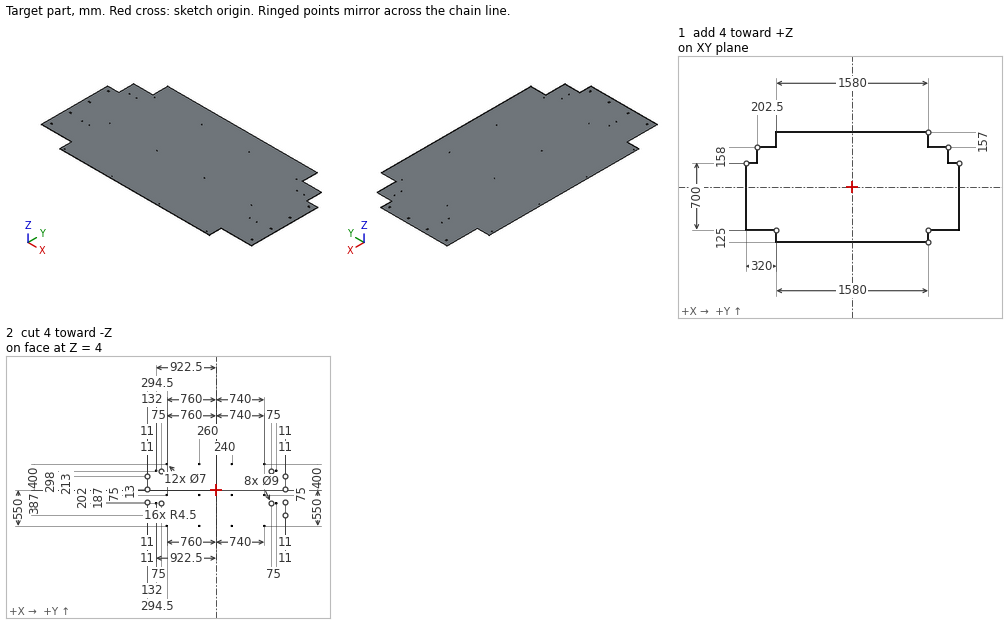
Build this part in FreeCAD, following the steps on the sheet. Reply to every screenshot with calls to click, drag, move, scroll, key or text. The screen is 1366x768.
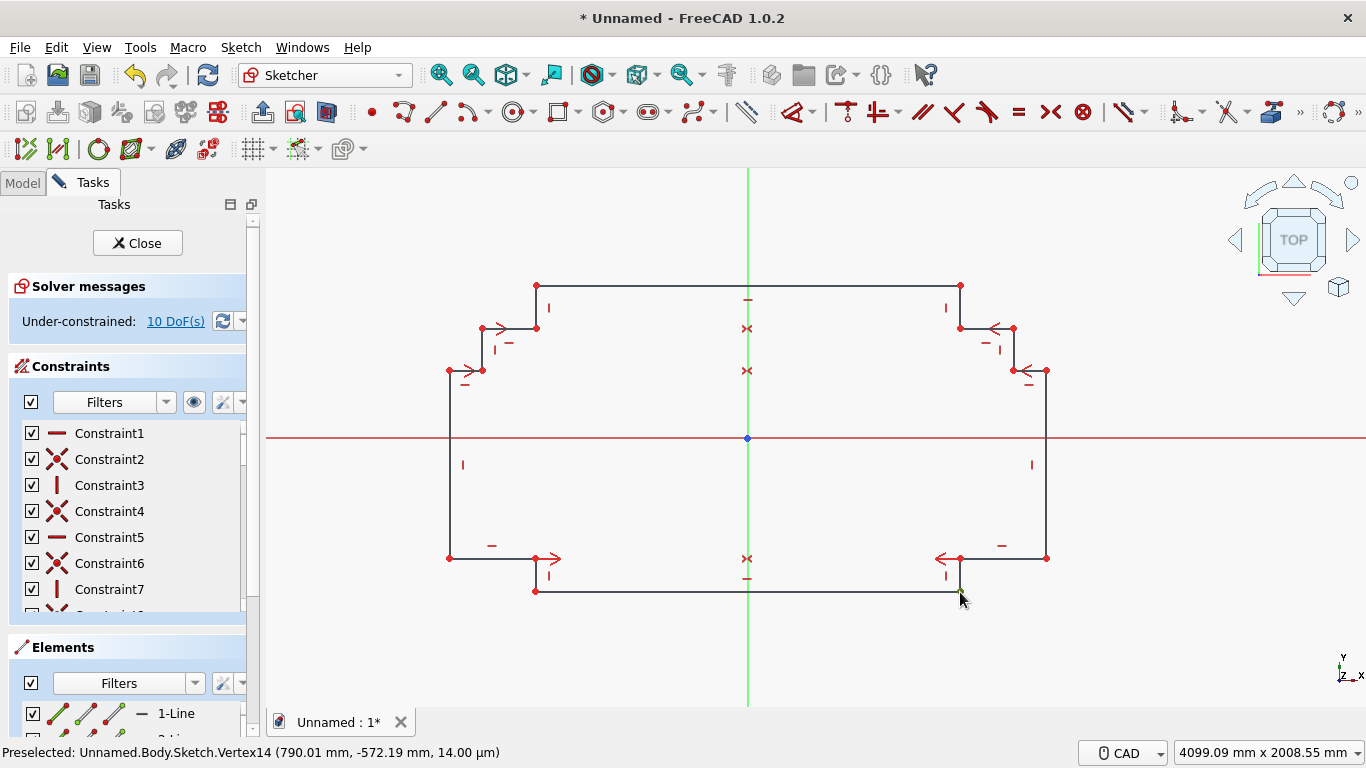
click(960, 286)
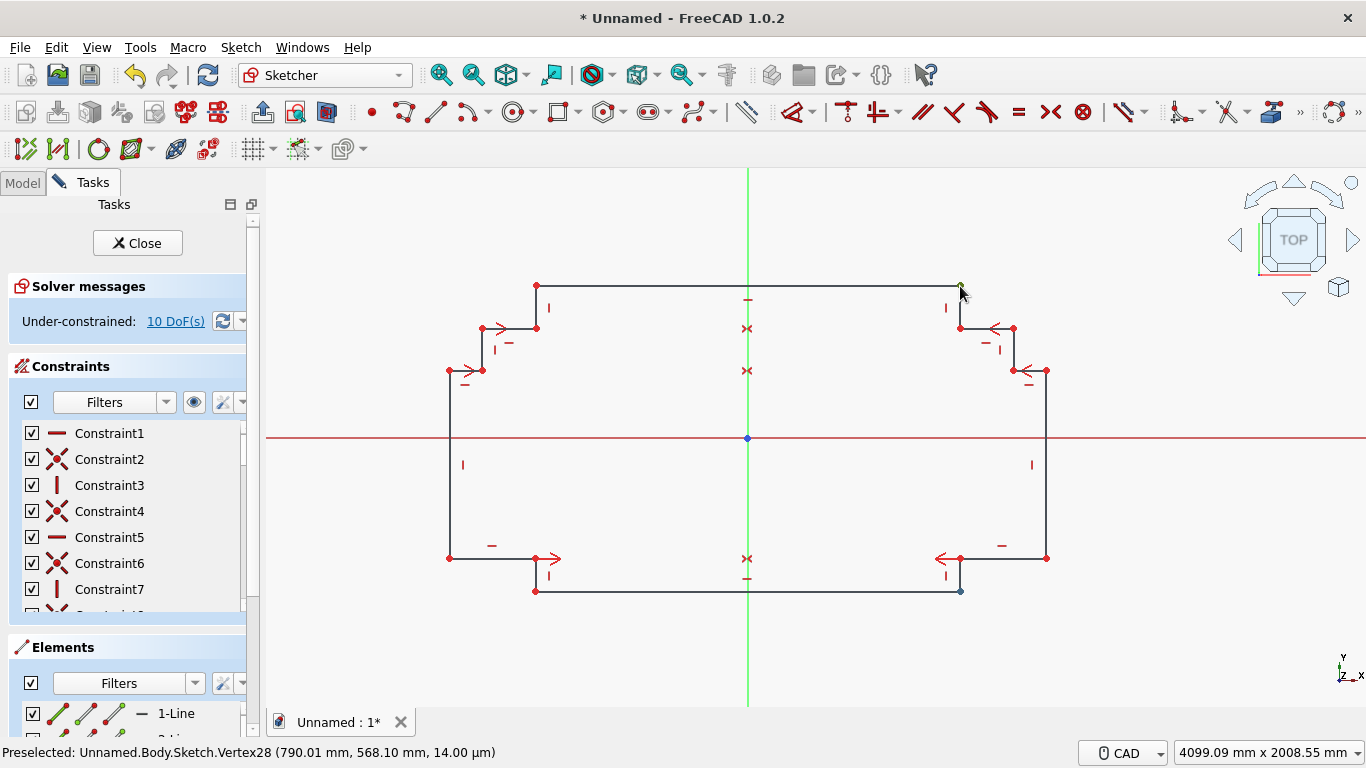
click(359, 438)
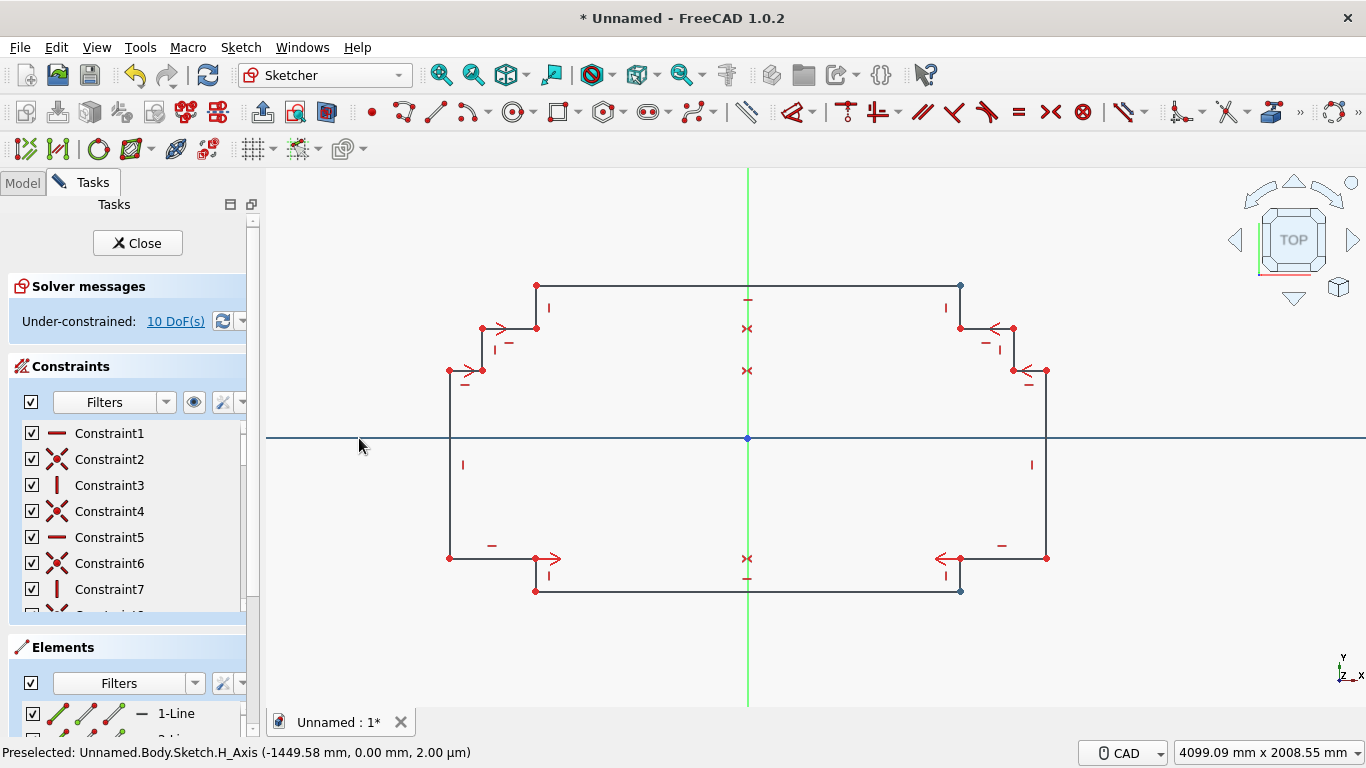
click(1052, 112)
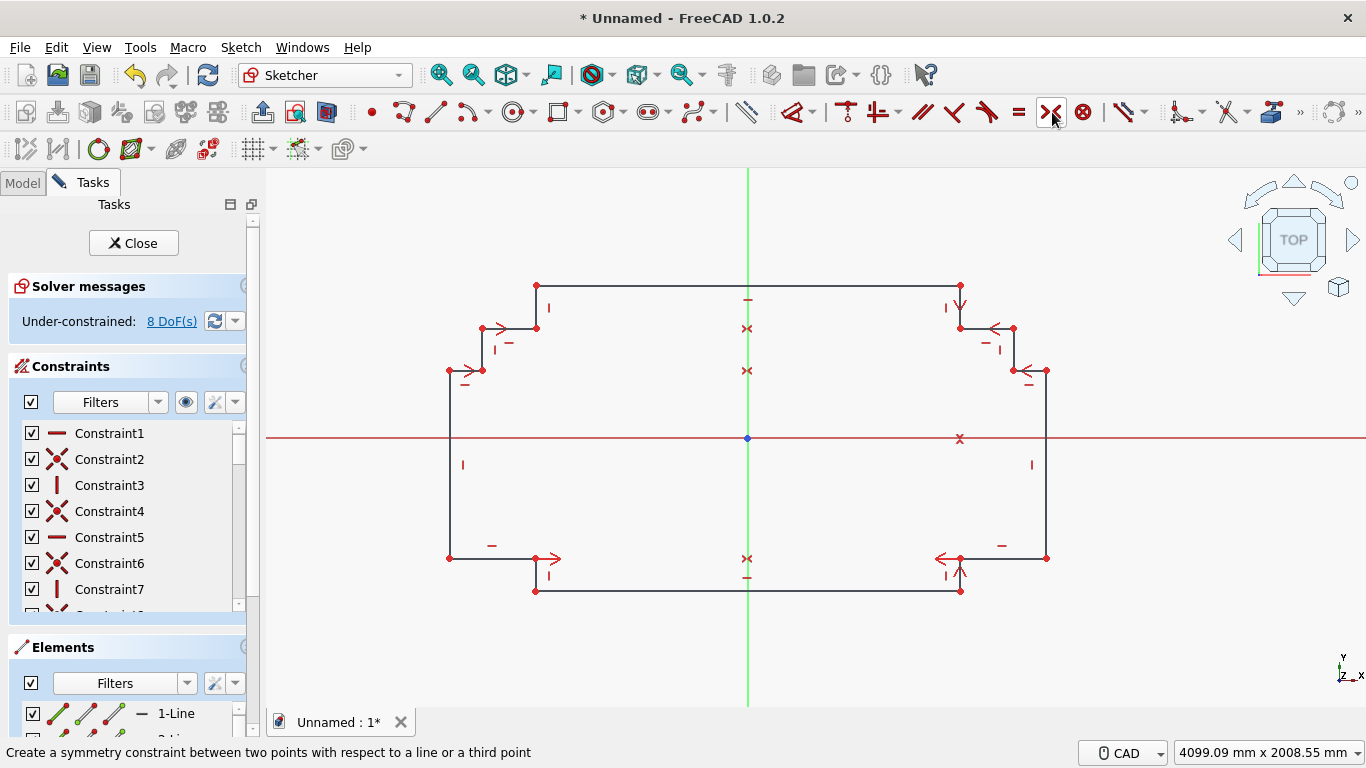
click(792, 112)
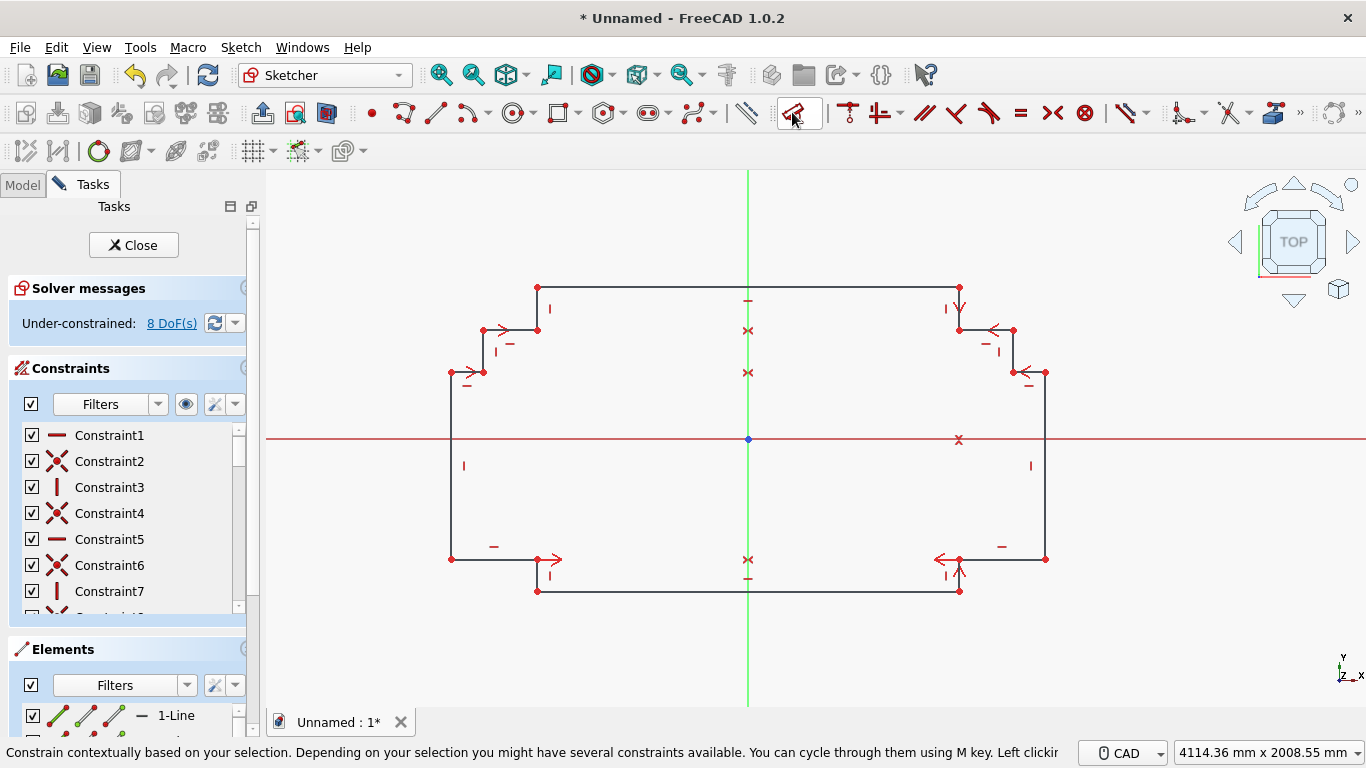
click(483, 343)
click(449, 351)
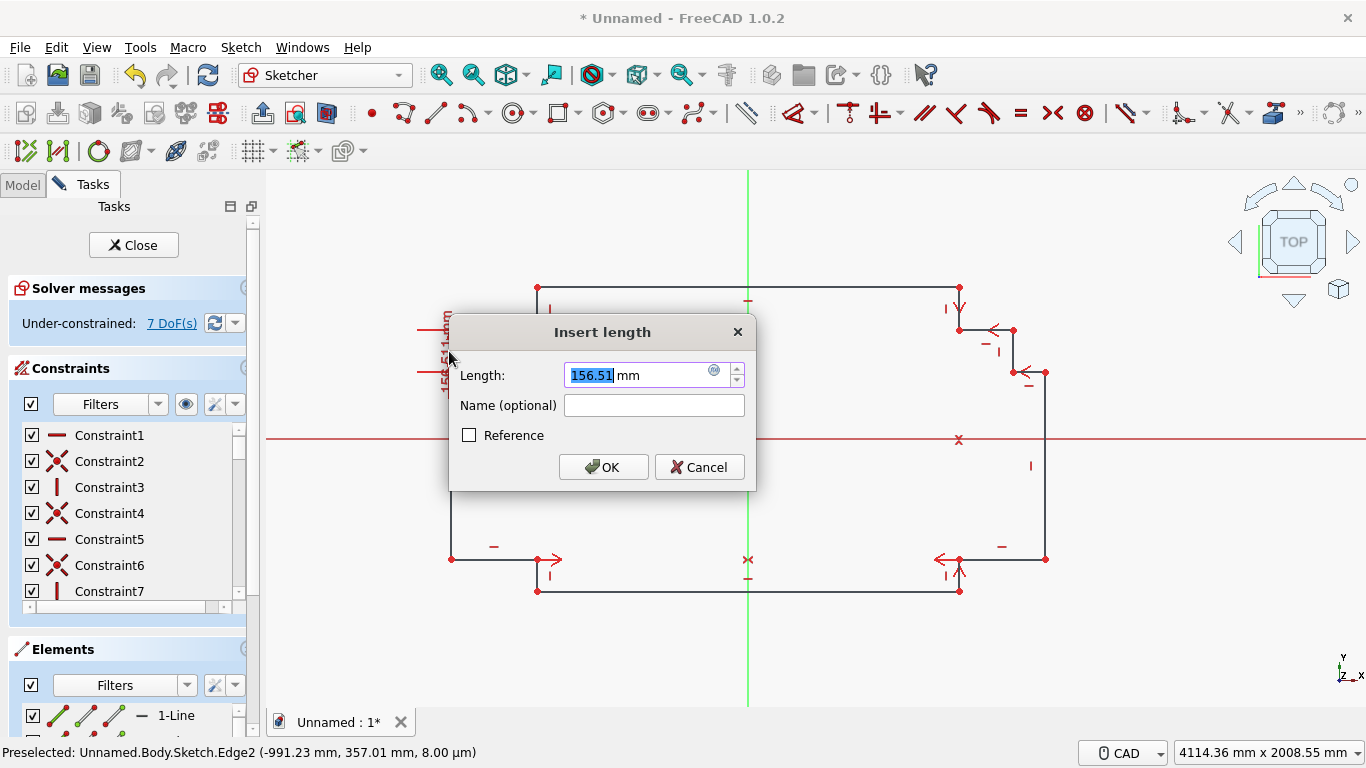
text(158)
key(Return)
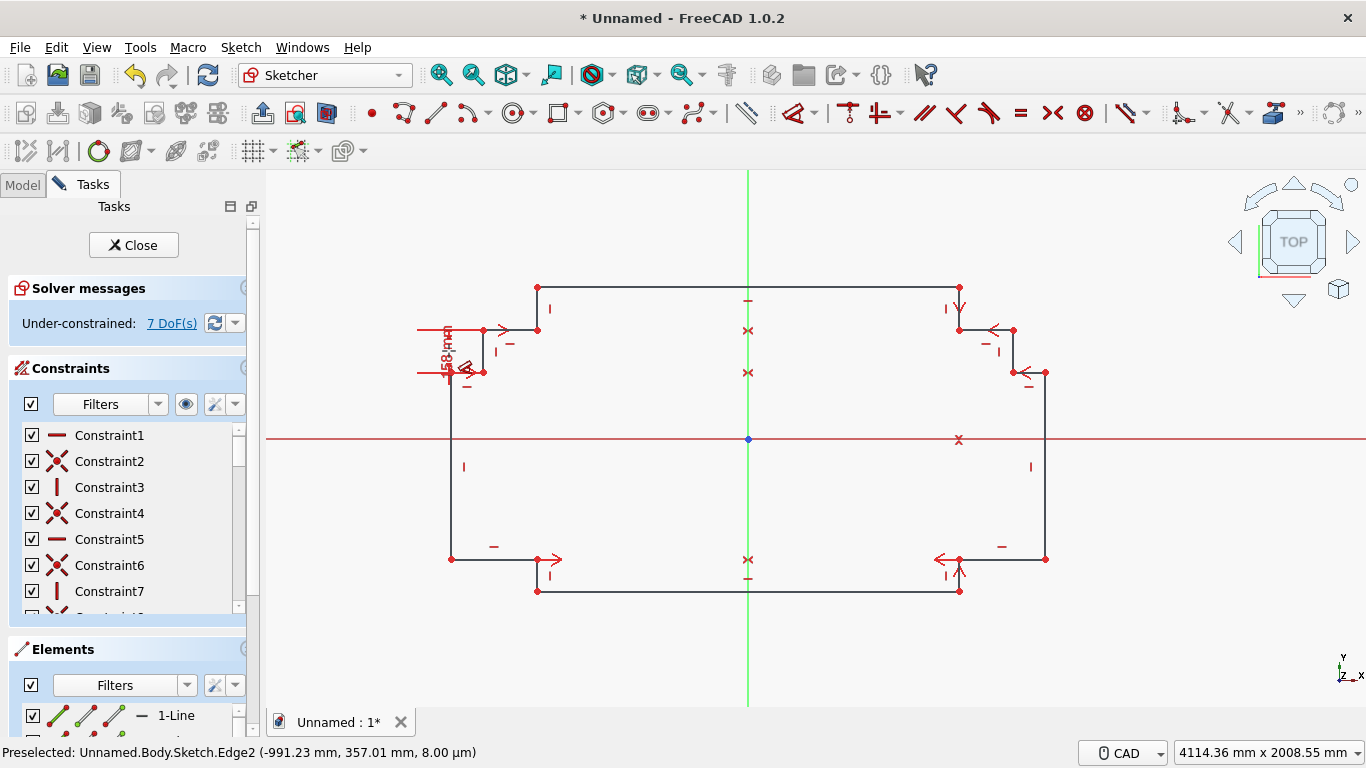
scroll(451, 429, up, 2)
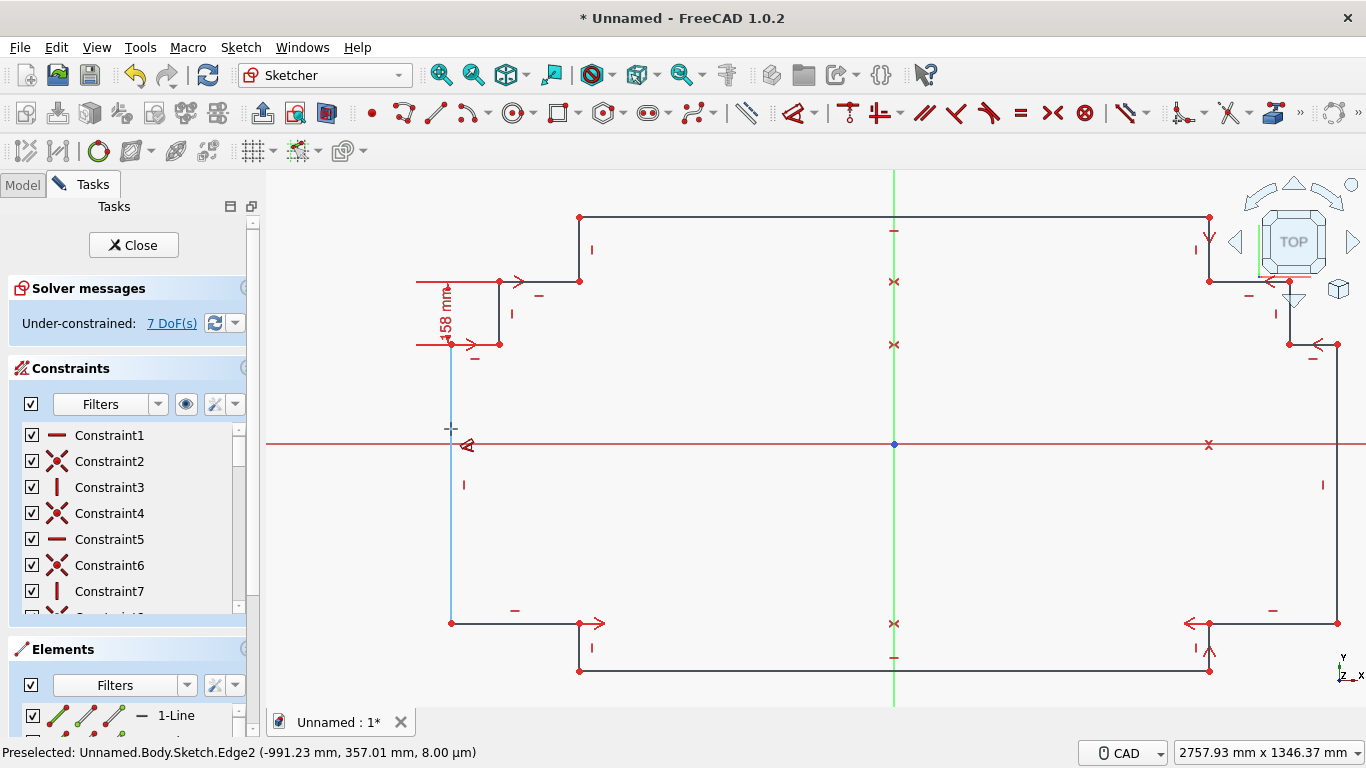
click(451, 428)
click(417, 484)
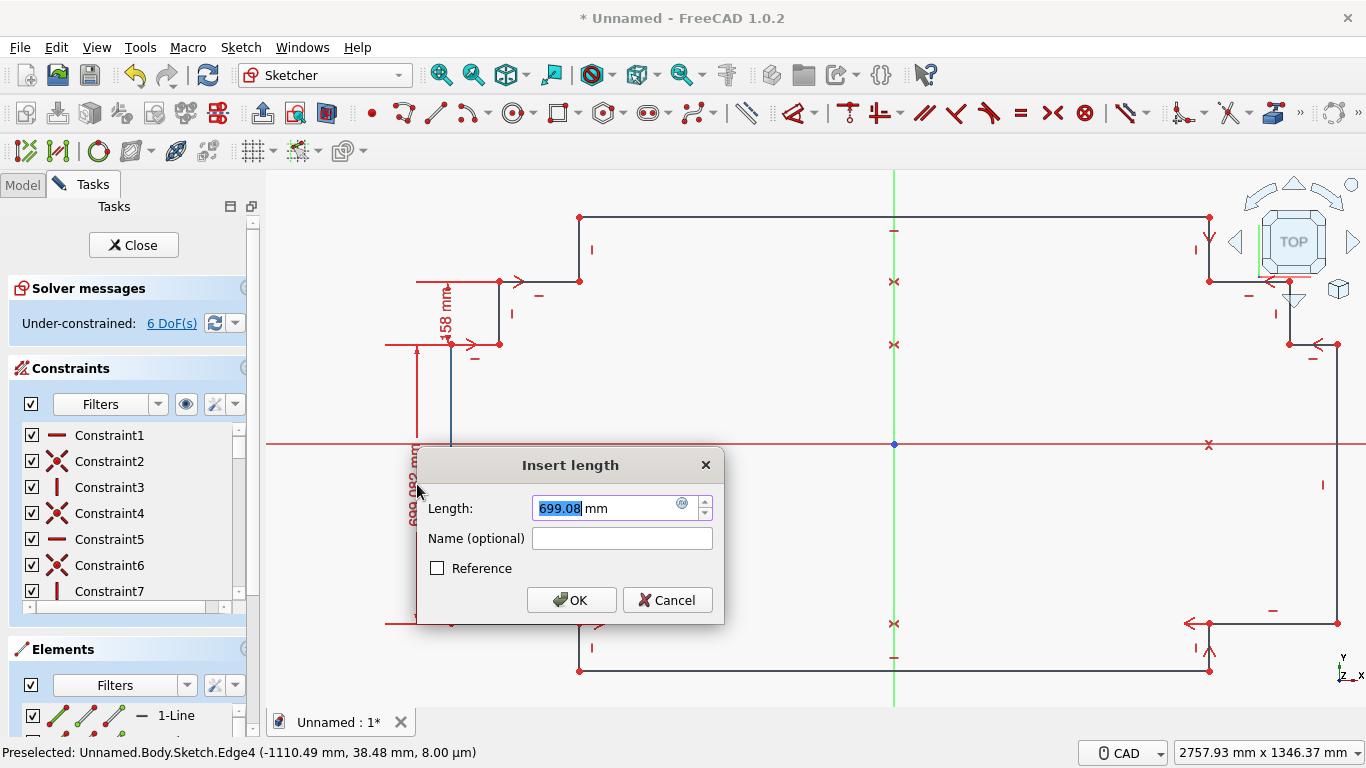
text(700)
key(Return)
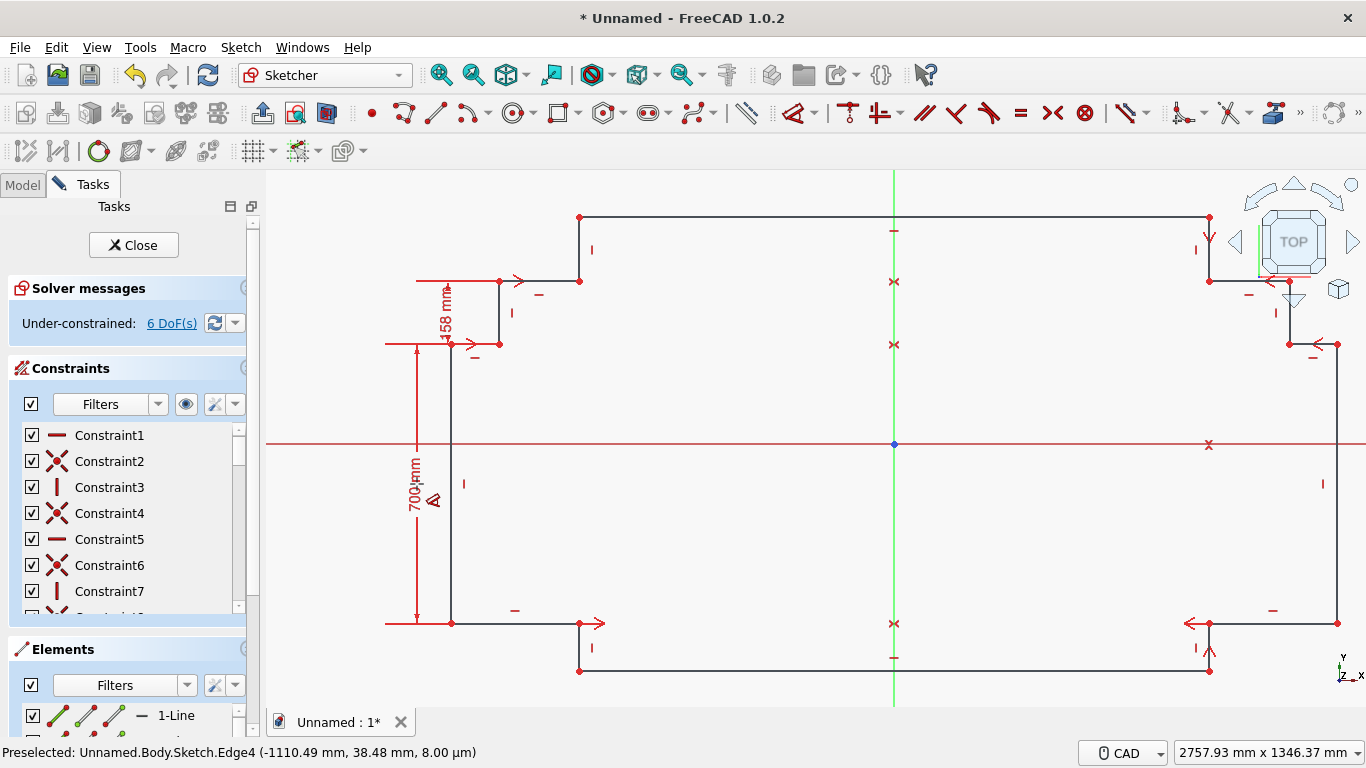
click(490, 624)
click(515, 658)